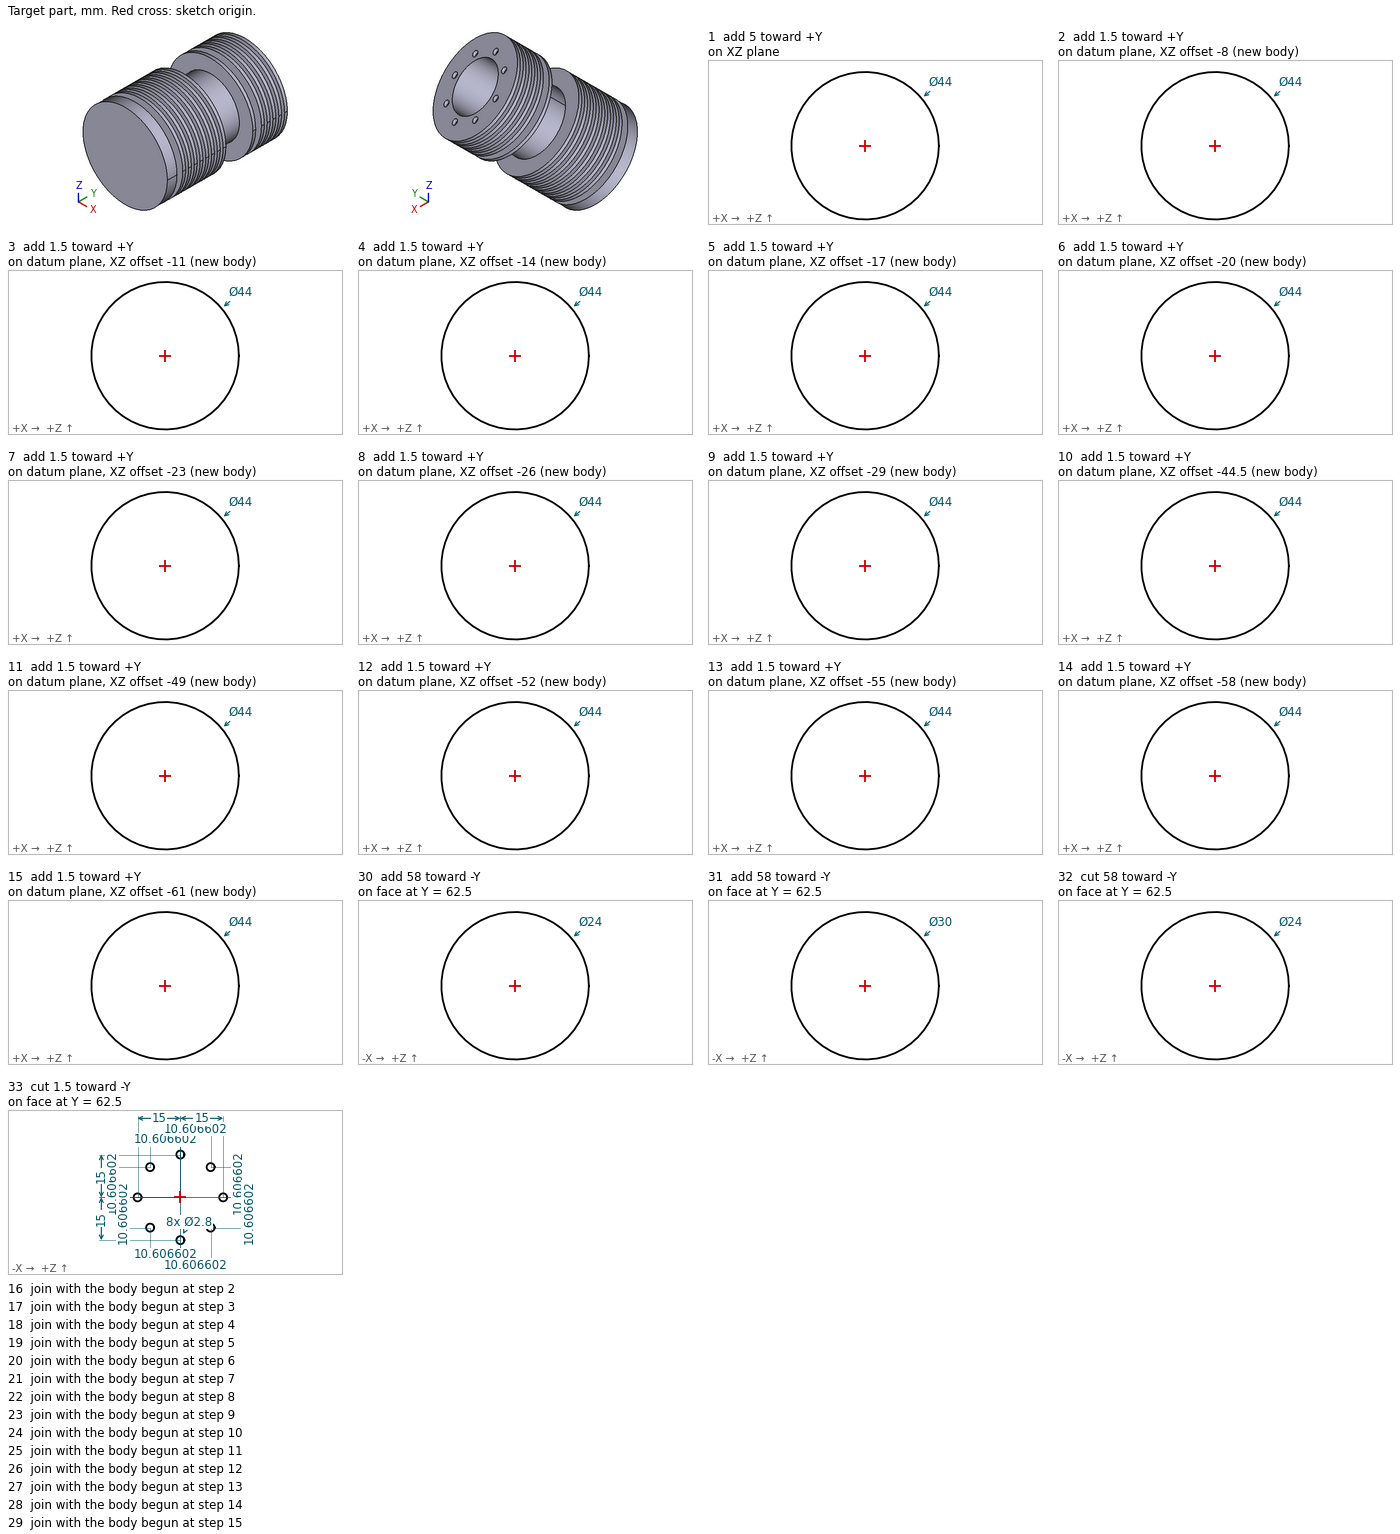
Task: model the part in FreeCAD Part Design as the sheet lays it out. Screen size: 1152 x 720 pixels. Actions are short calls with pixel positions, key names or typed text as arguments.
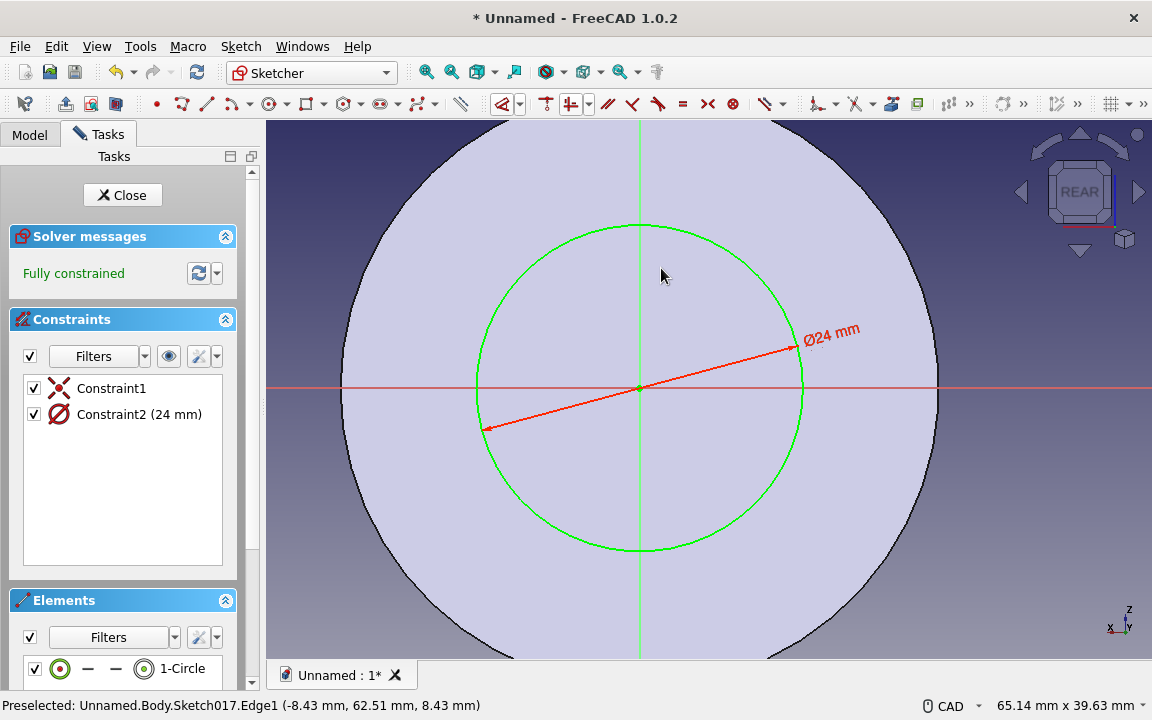
click(123, 195)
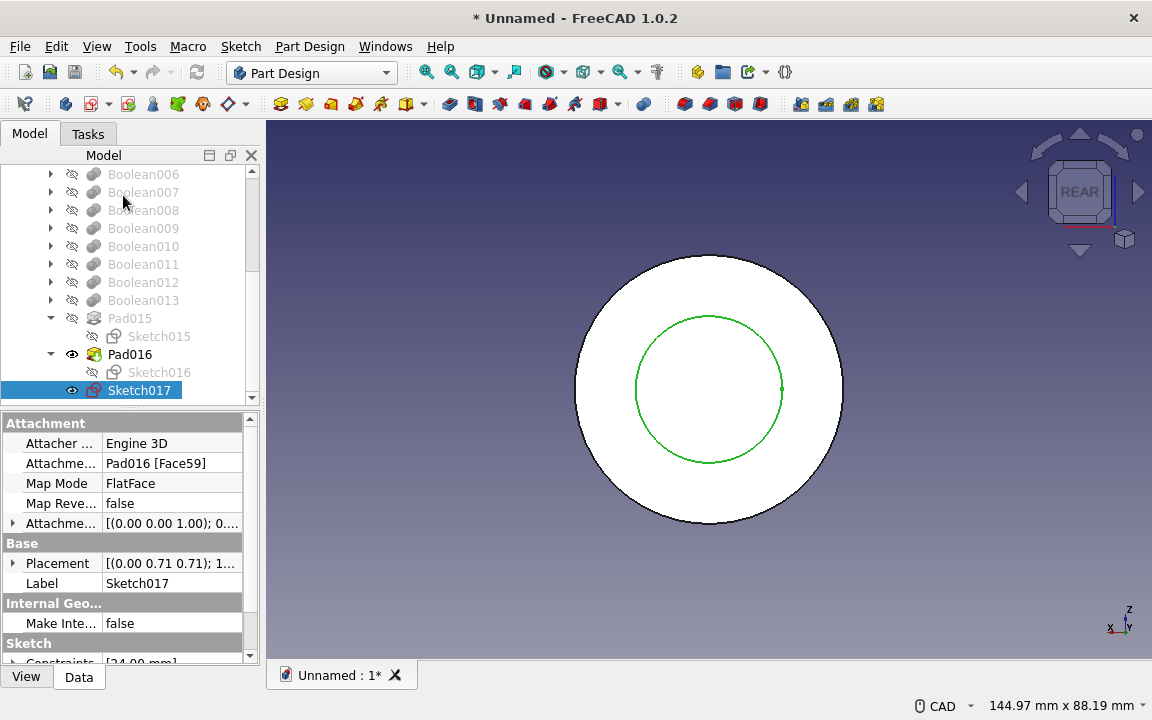
click(450, 104)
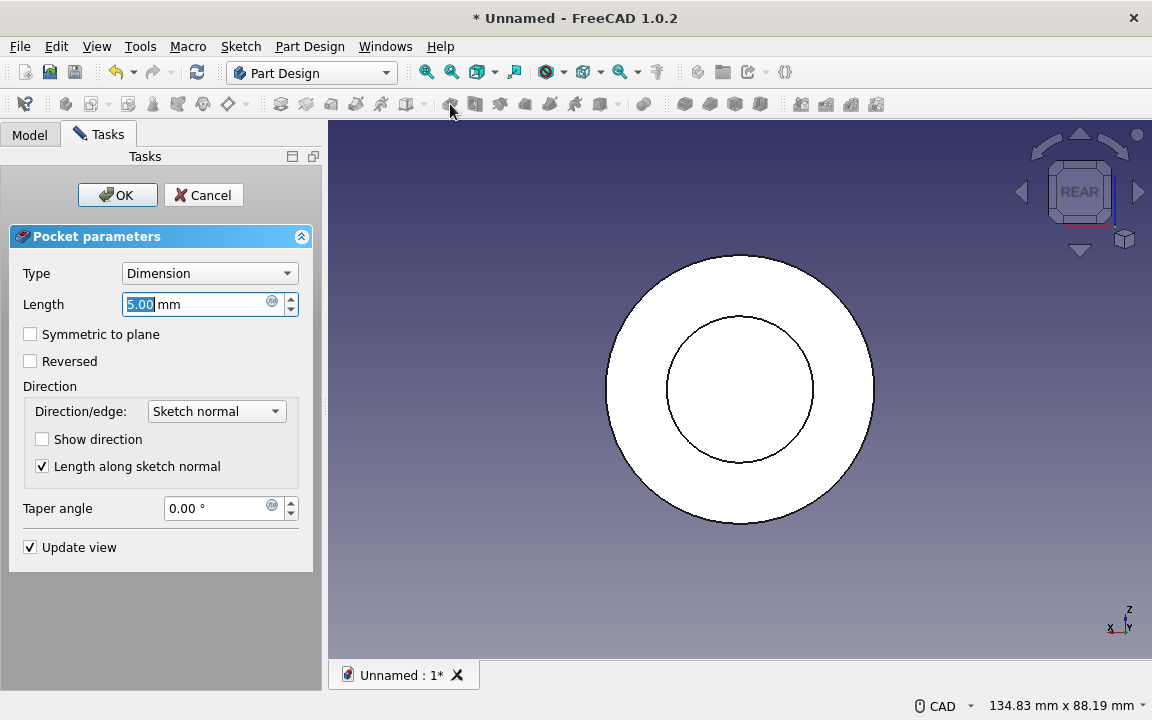
text(58)
key(Tab)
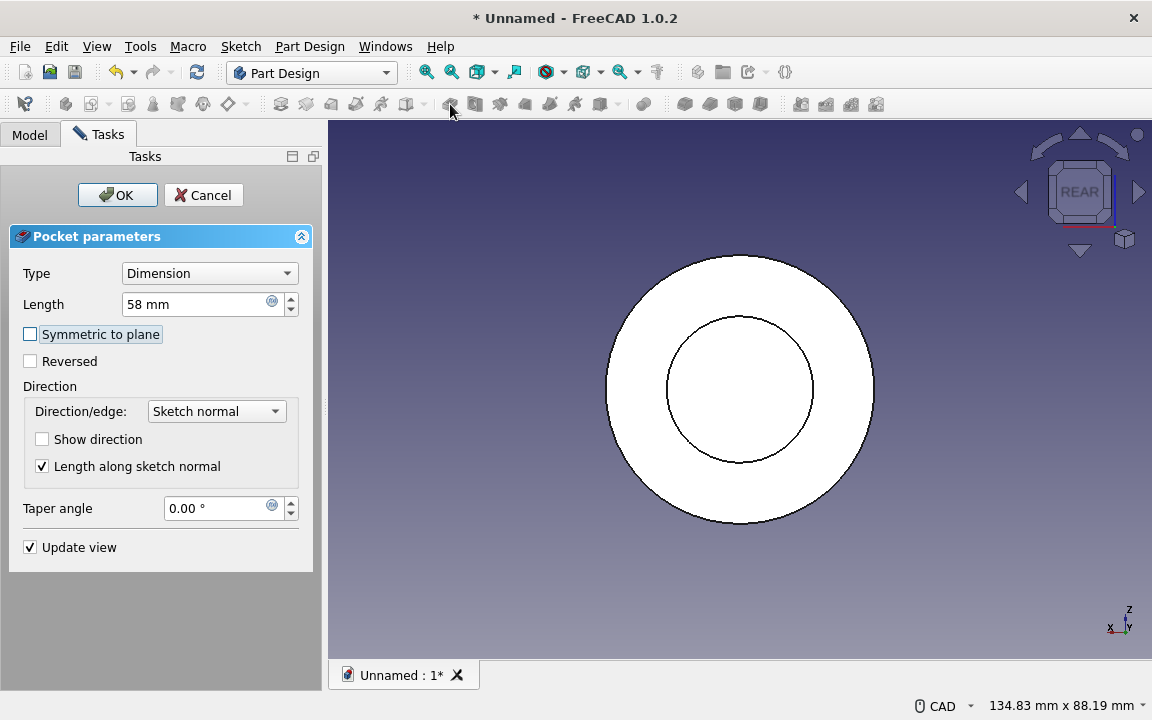
click(118, 195)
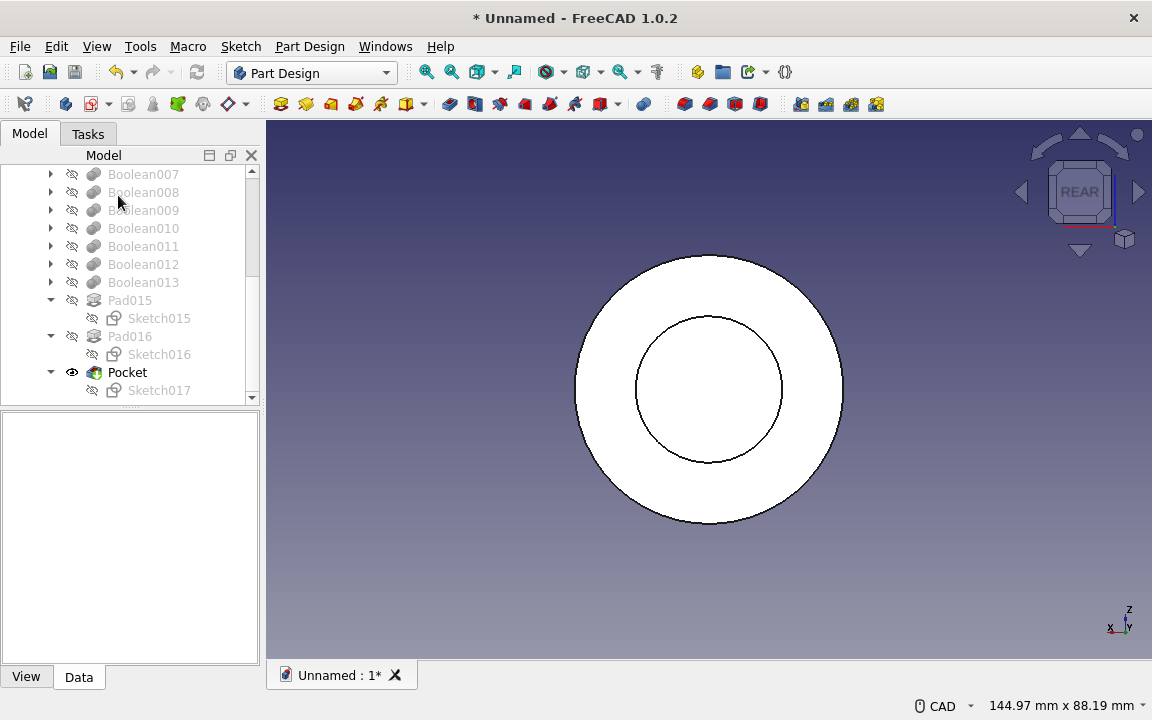
click(632, 312)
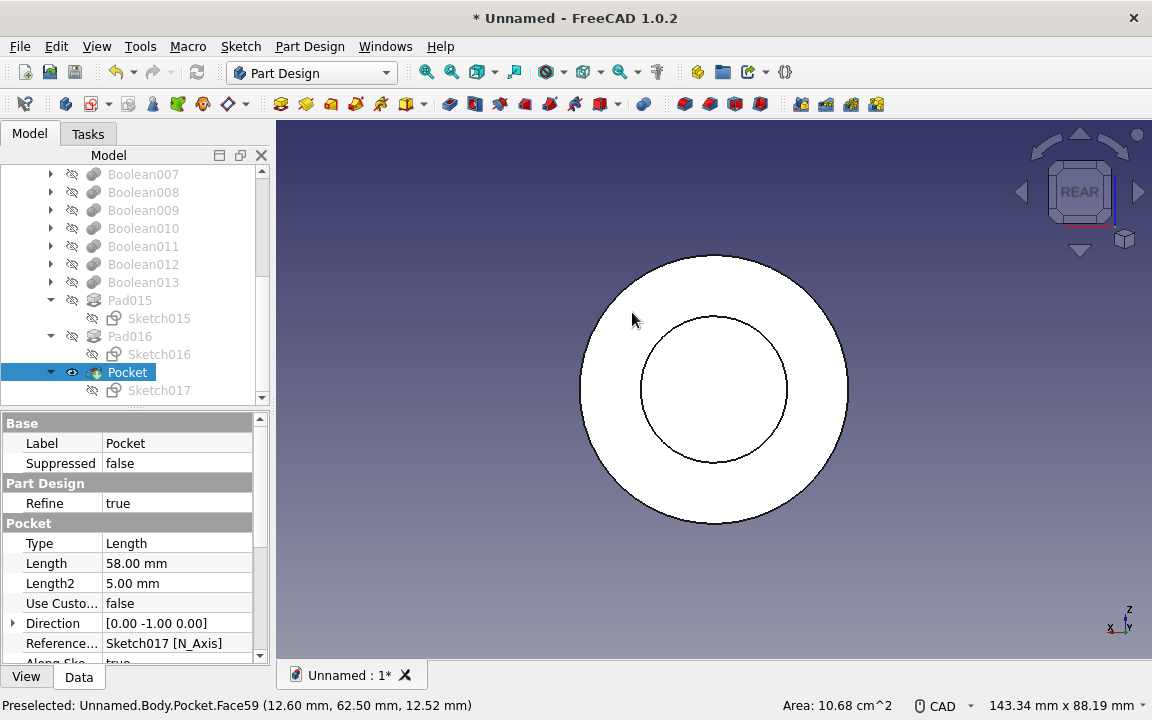
click(90, 104)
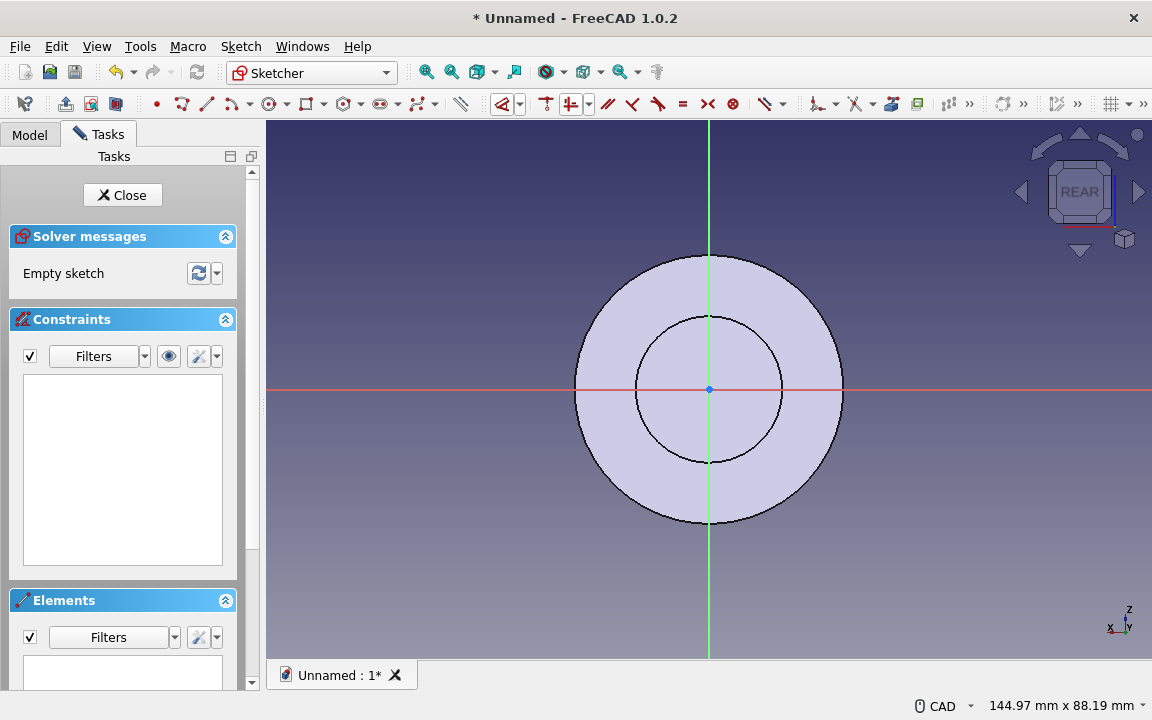
scroll(792, 390, up, 3)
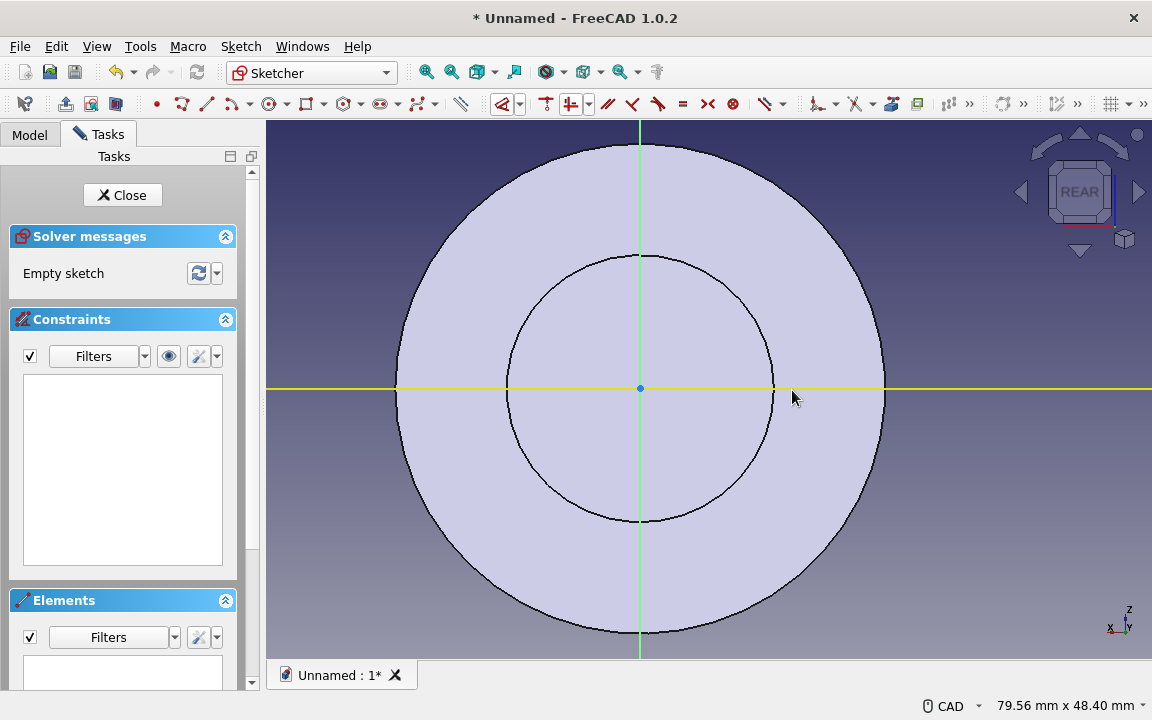
key(g)
key(c)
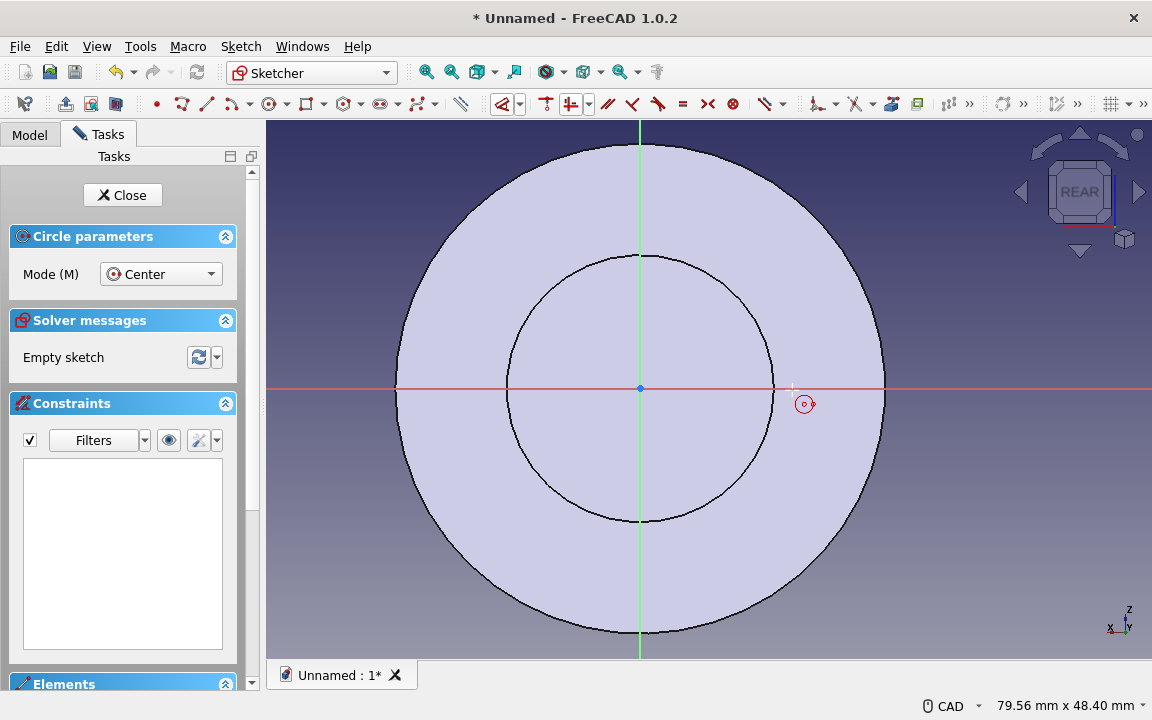
scroll(640, 556, up, 2)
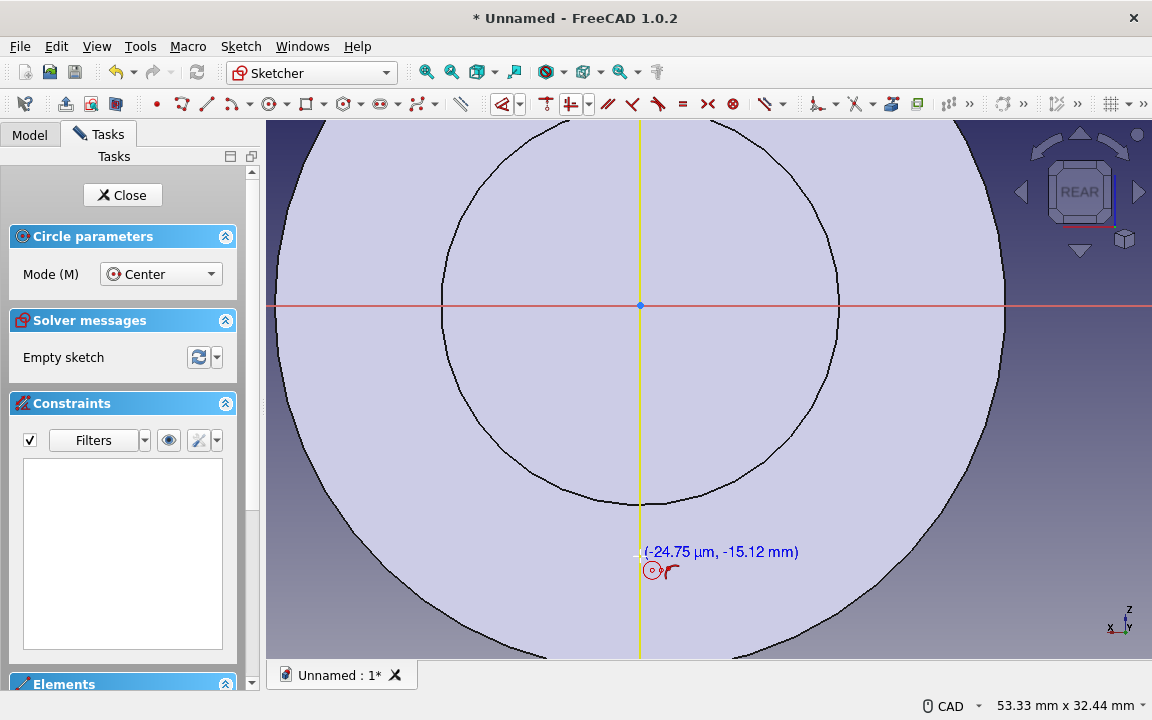
click(640, 555)
click(657, 539)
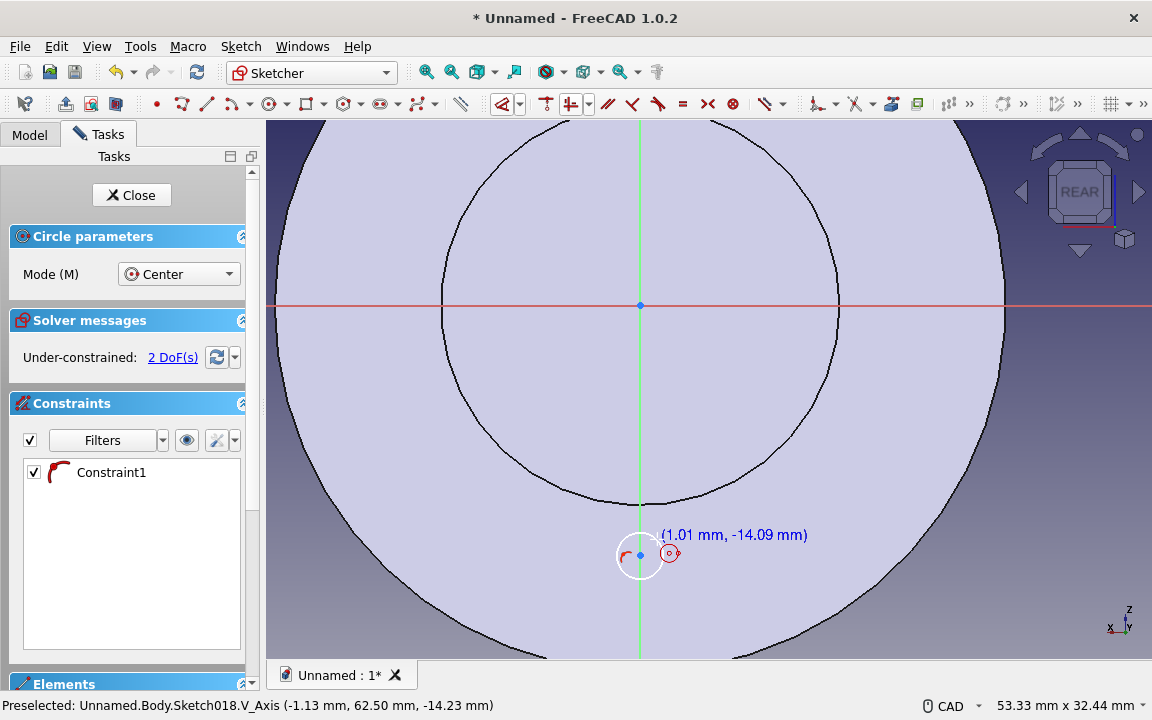
click(464, 482)
click(480, 466)